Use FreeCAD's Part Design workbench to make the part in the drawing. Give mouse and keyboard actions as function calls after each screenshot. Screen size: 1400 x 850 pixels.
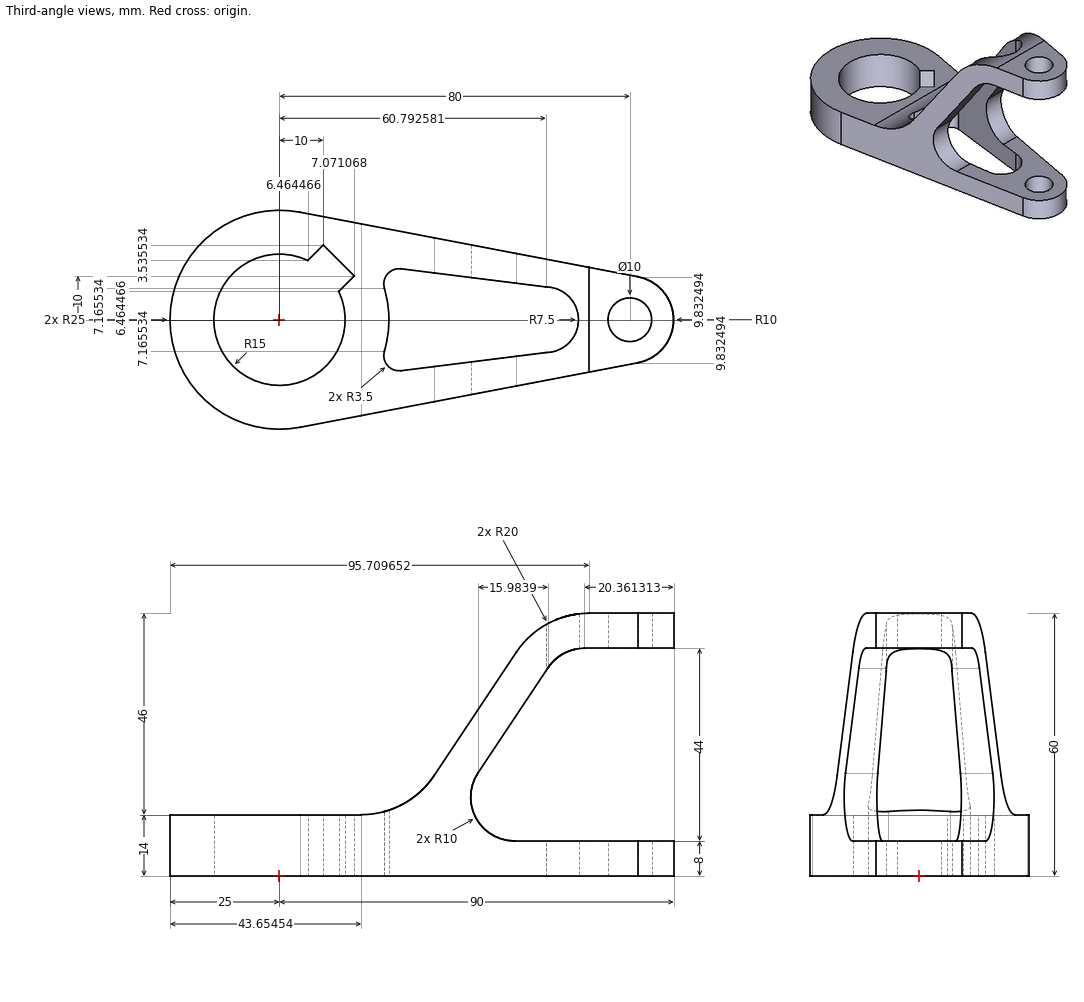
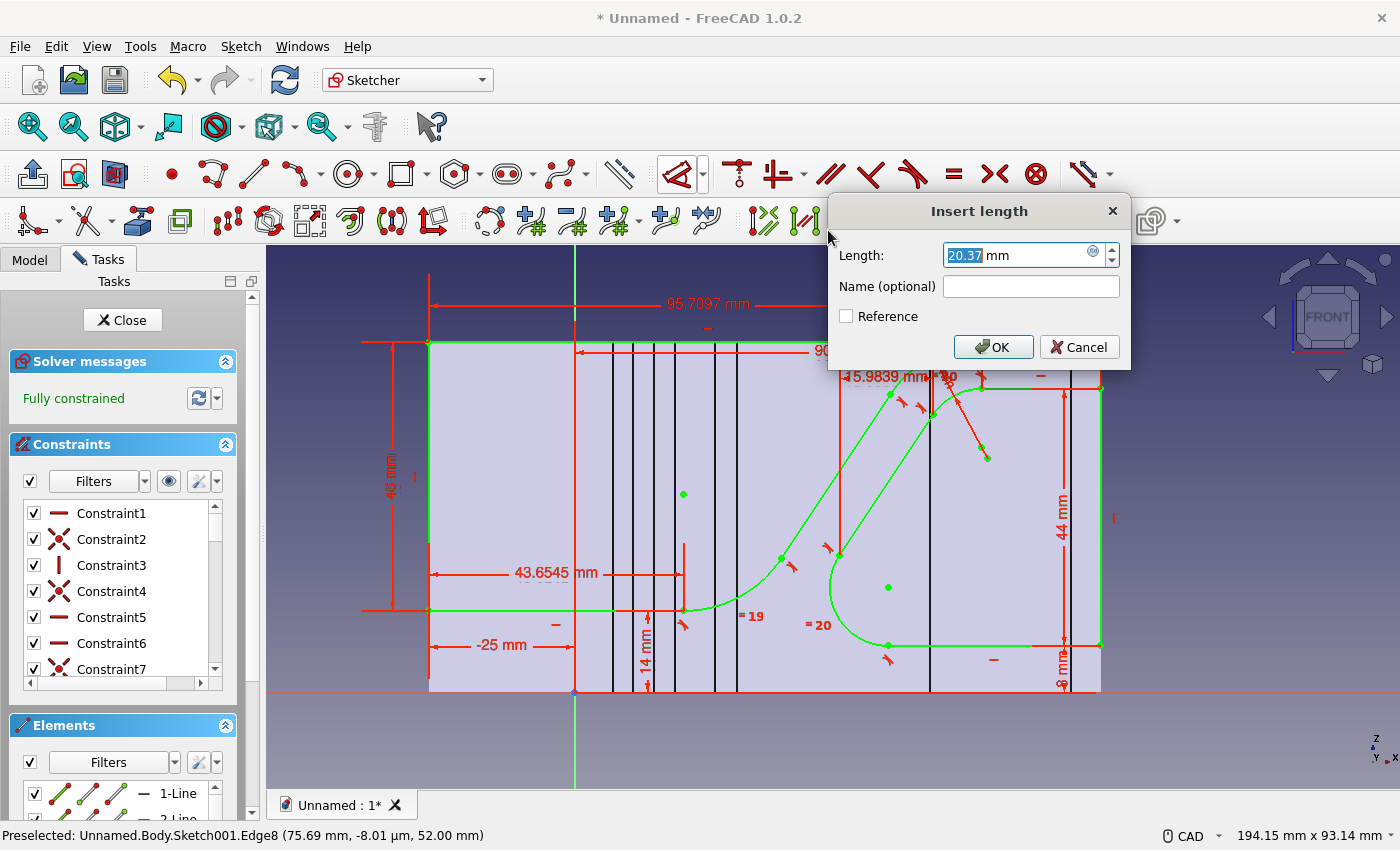
text(20.361313)
key(Return)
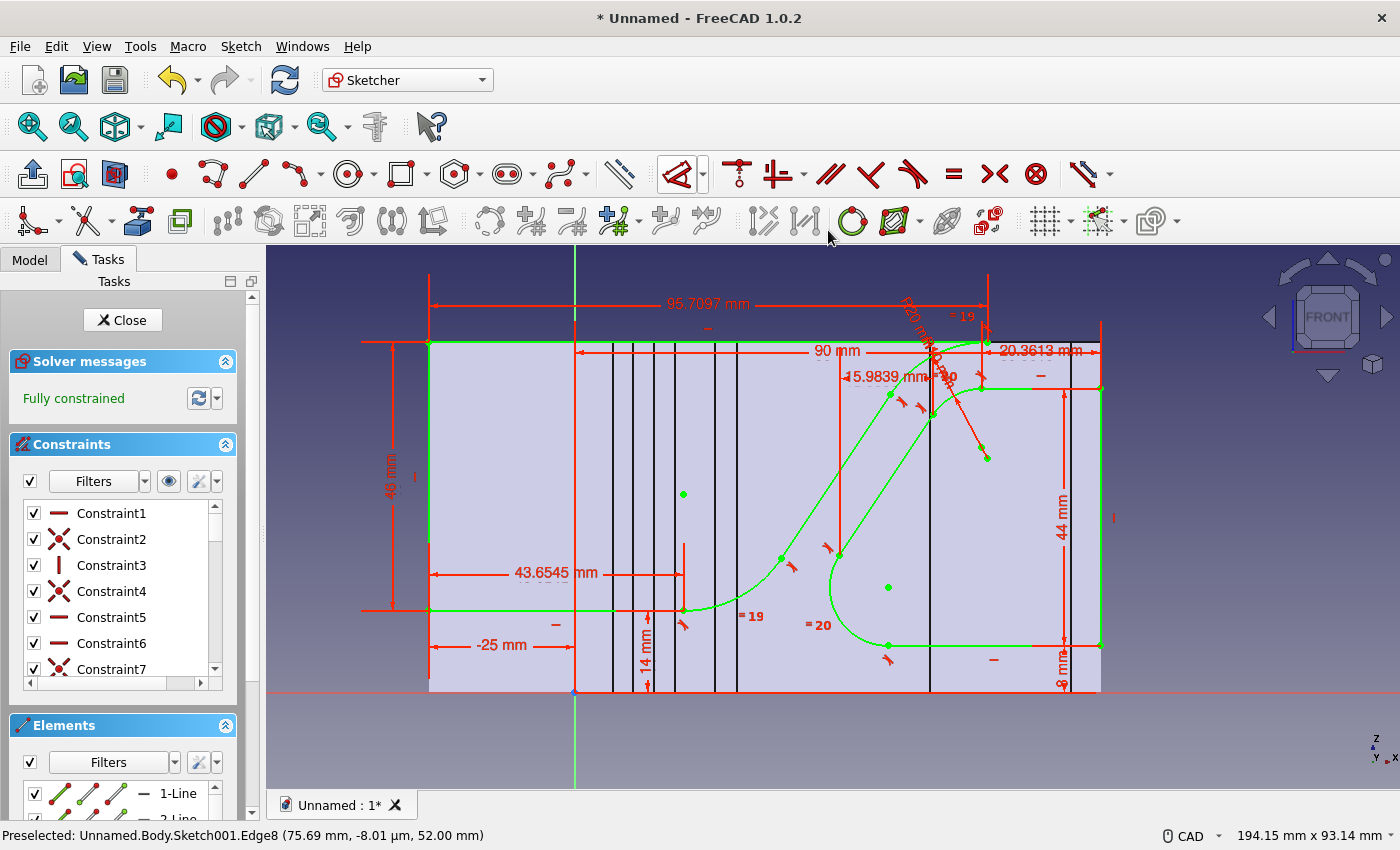
click(123, 320)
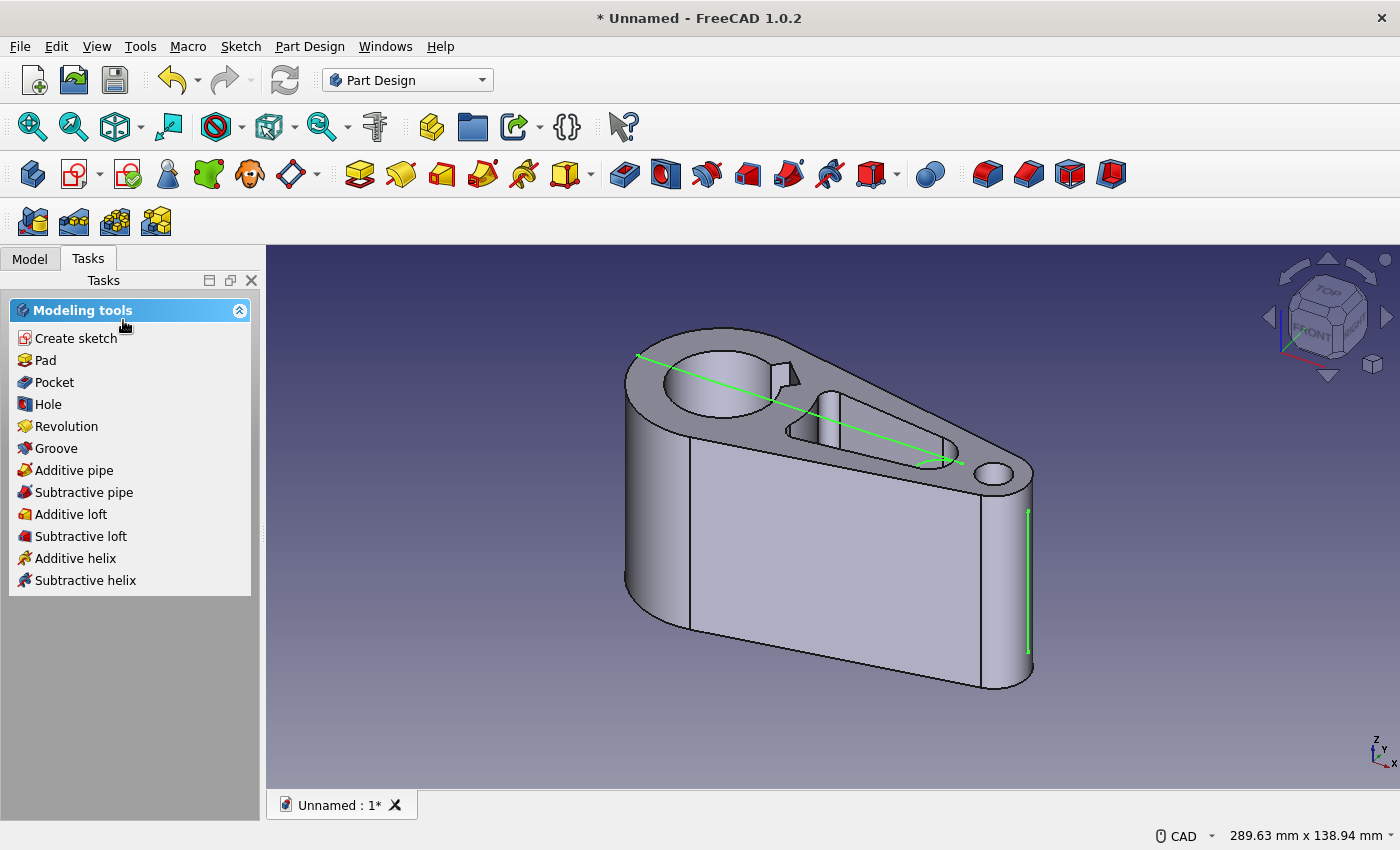
click(625, 174)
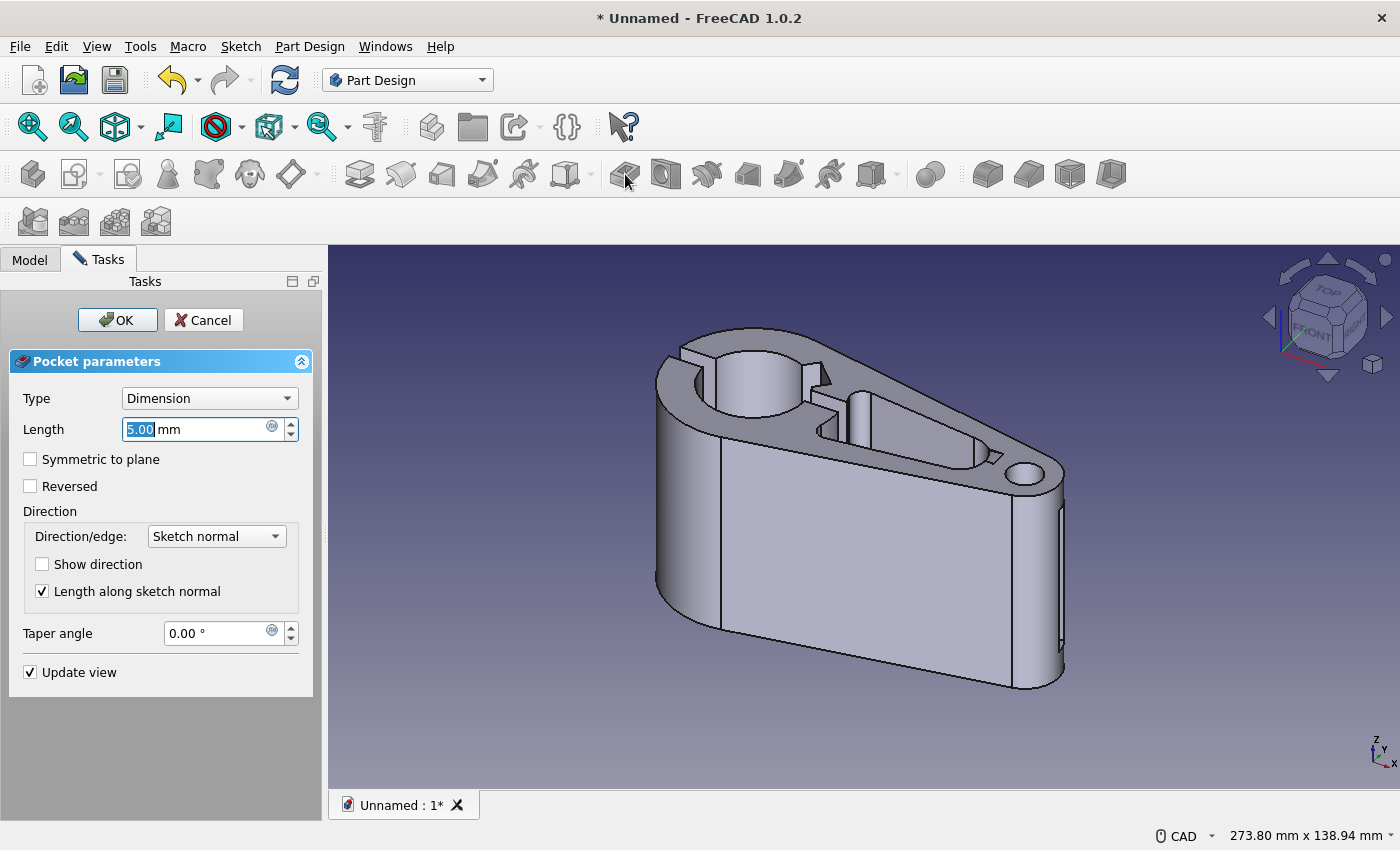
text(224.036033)
key(Tab)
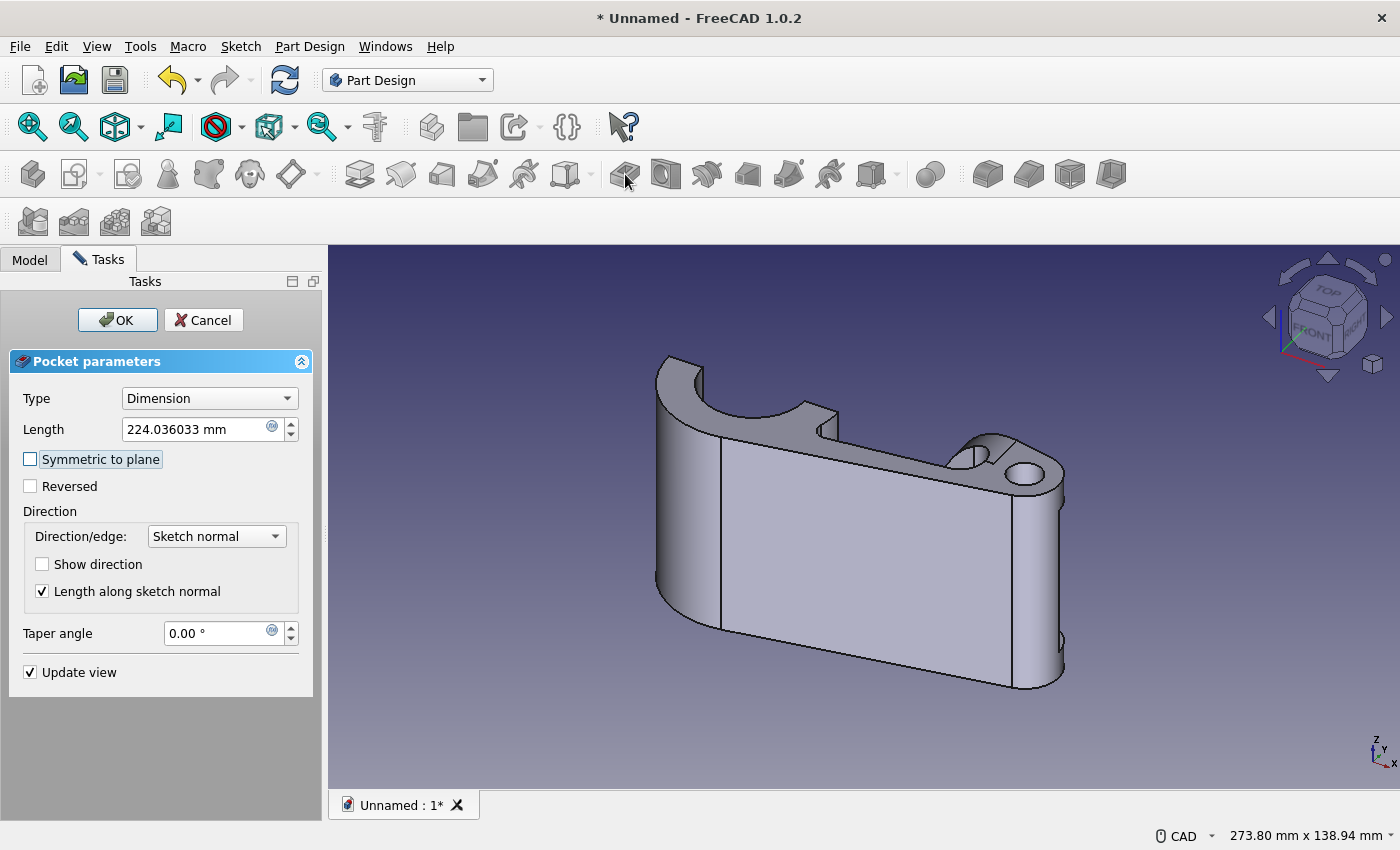
click(31, 459)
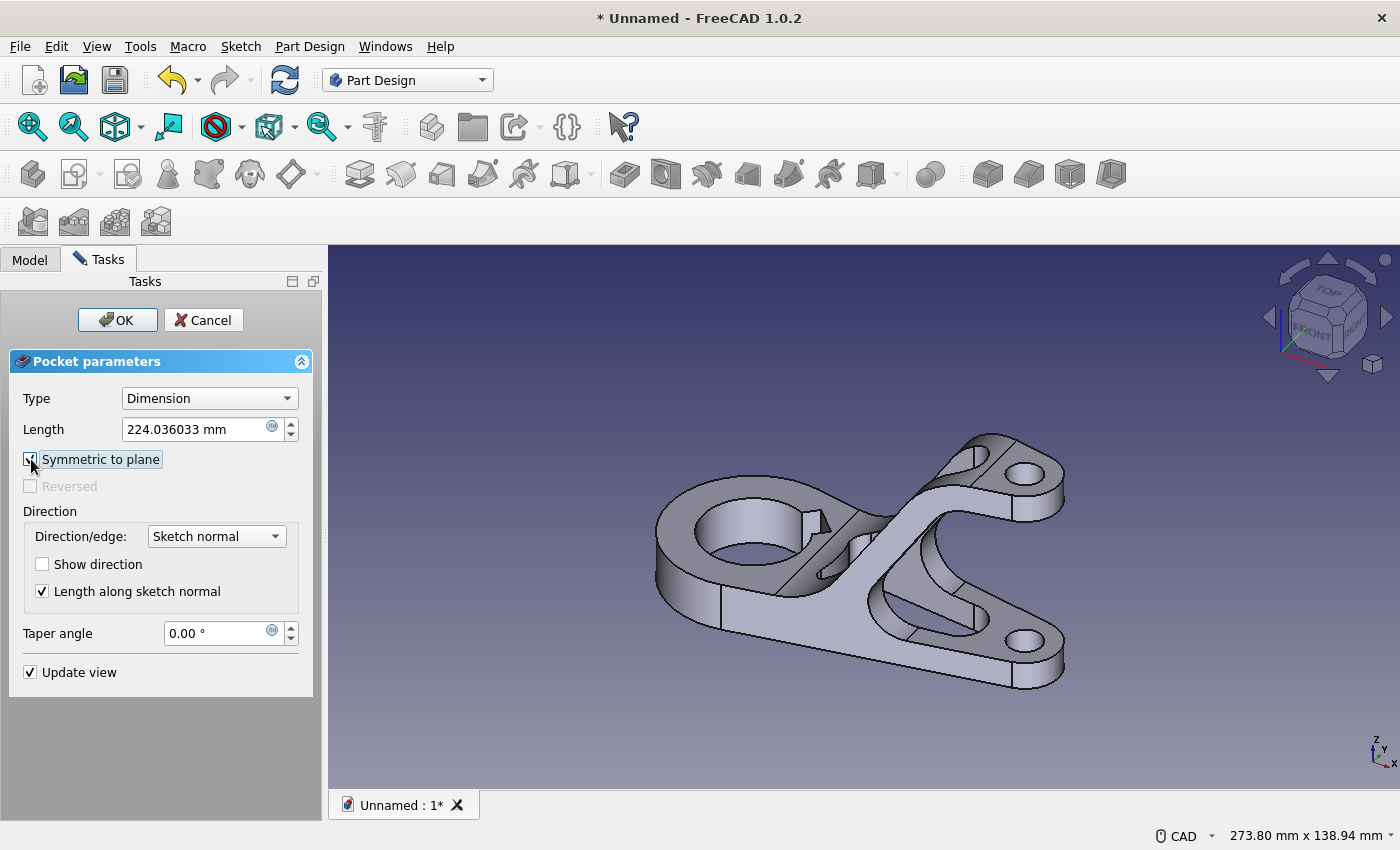
click(118, 320)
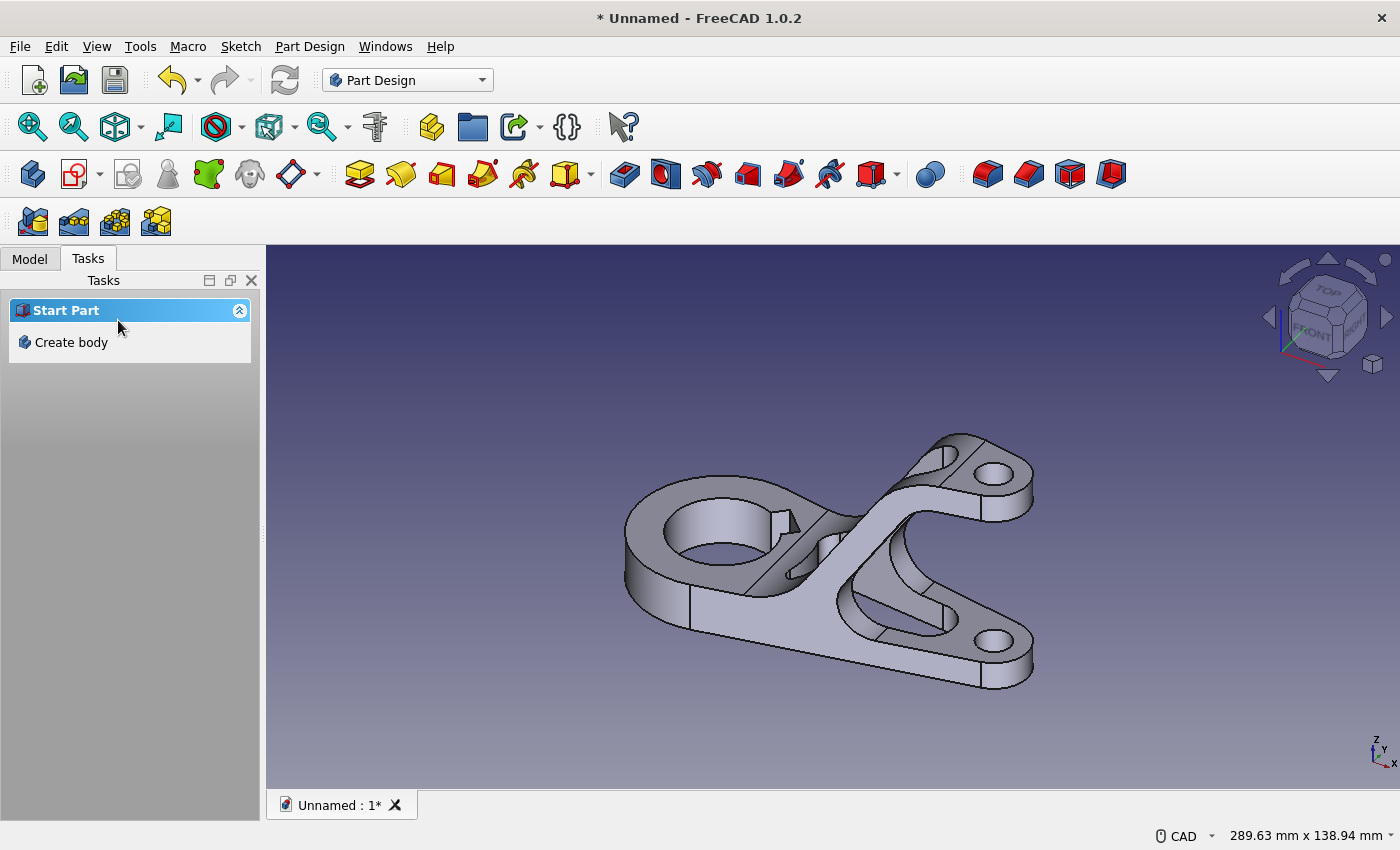
key(0)